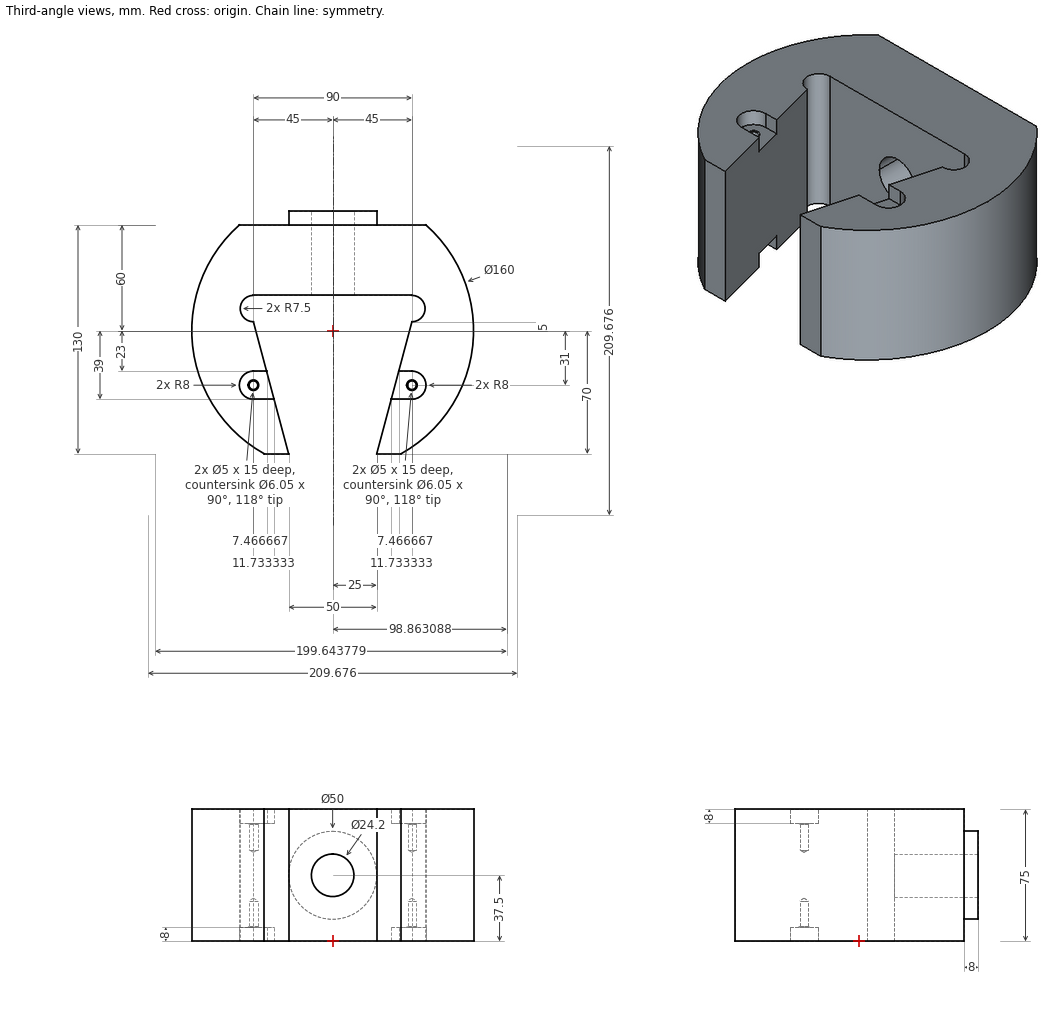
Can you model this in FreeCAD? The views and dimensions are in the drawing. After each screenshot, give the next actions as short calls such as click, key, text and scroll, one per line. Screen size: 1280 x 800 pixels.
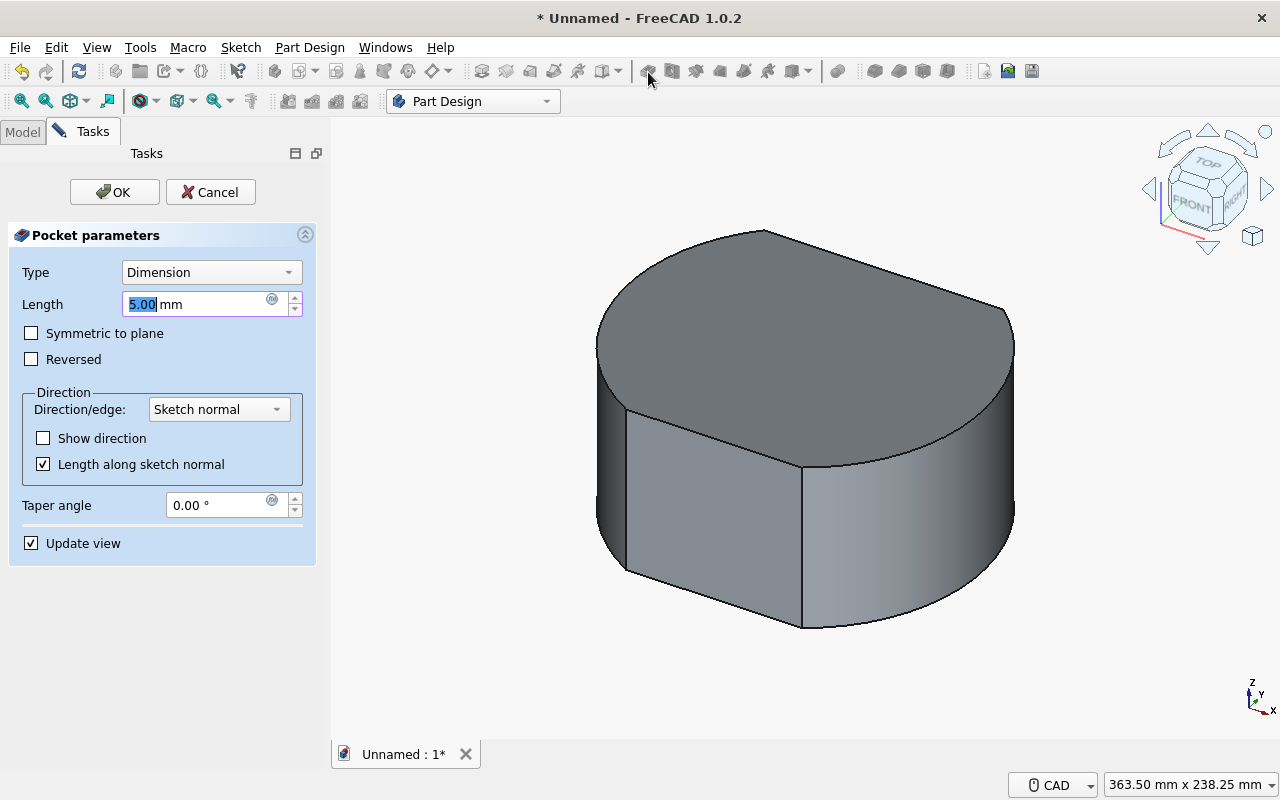
click(212, 272)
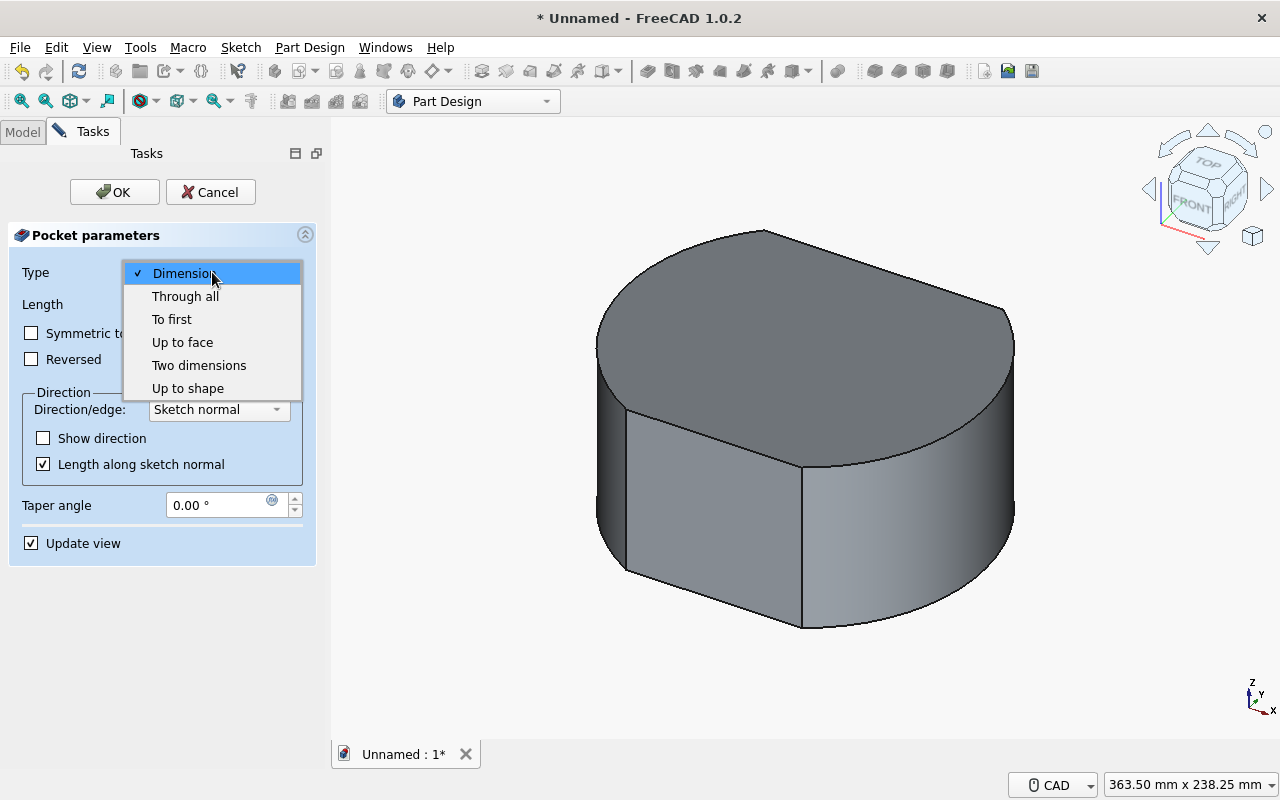
click(212, 296)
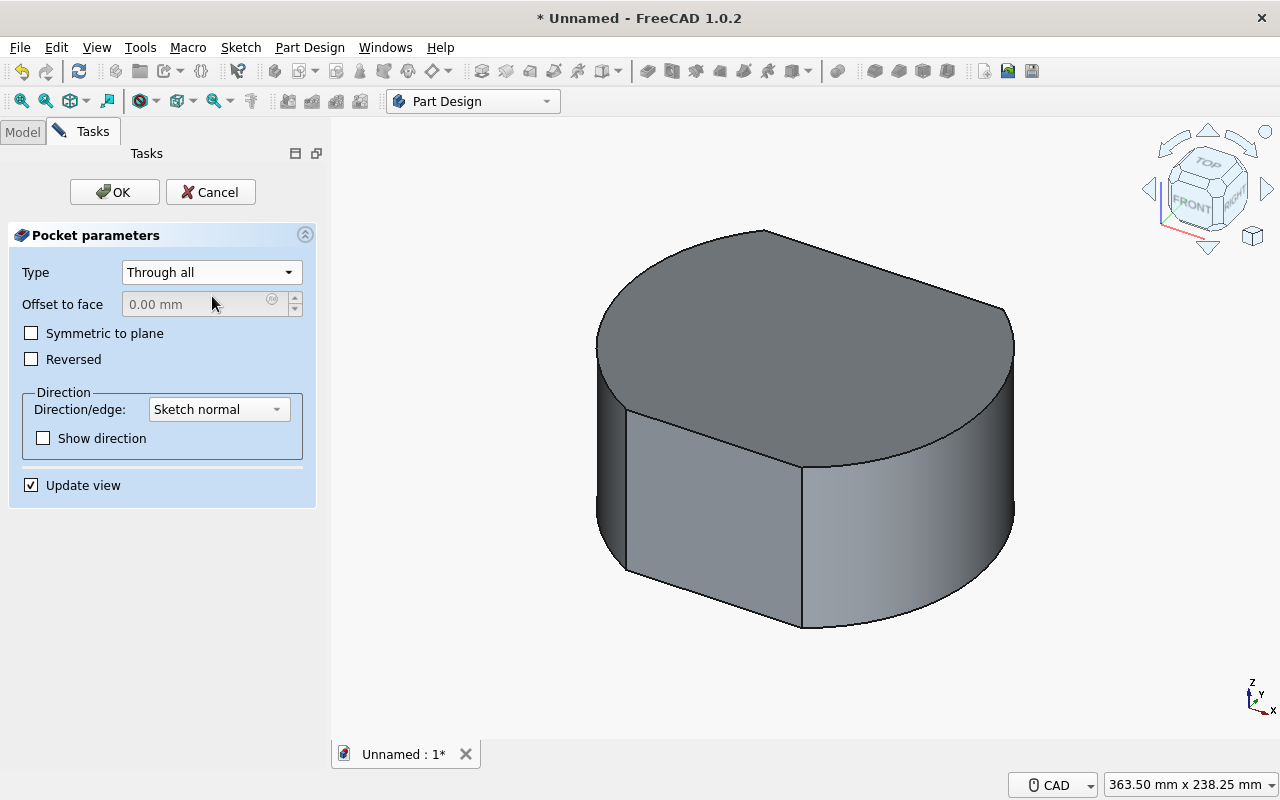
click(30, 359)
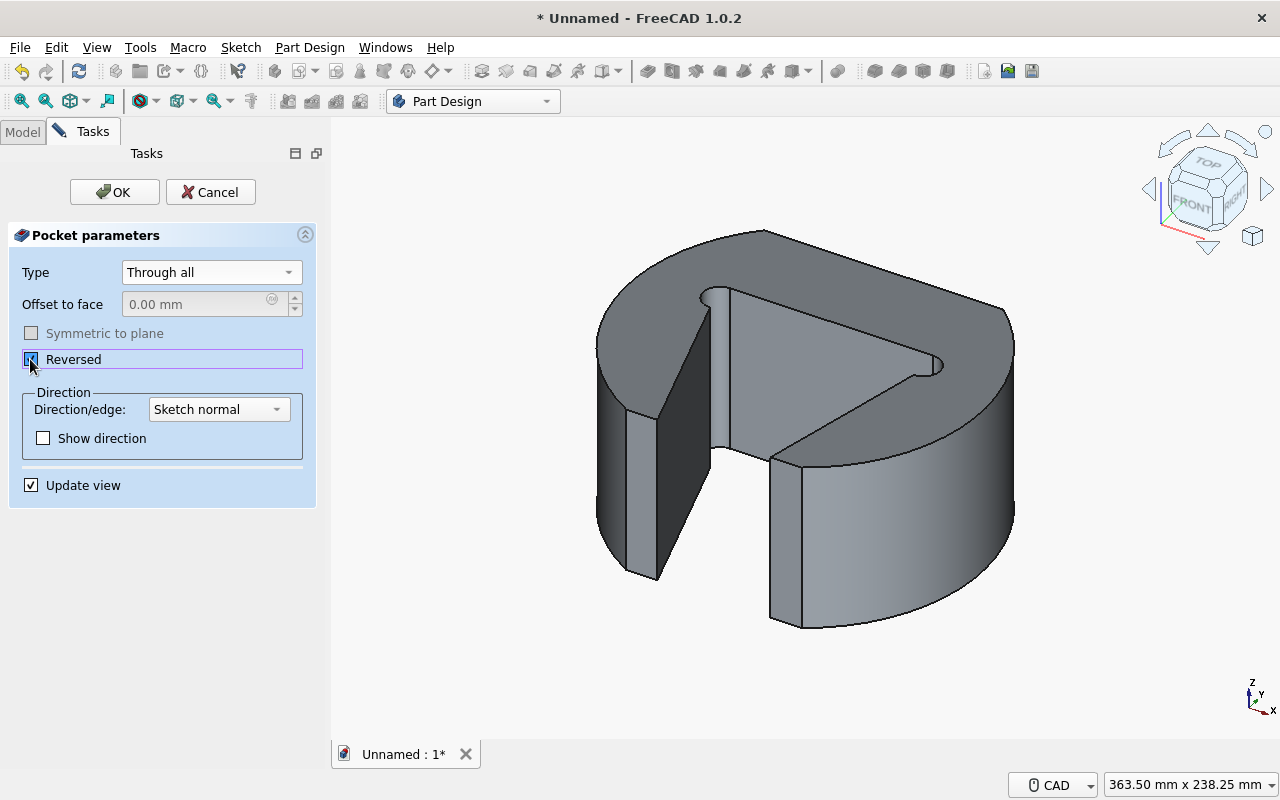
click(115, 192)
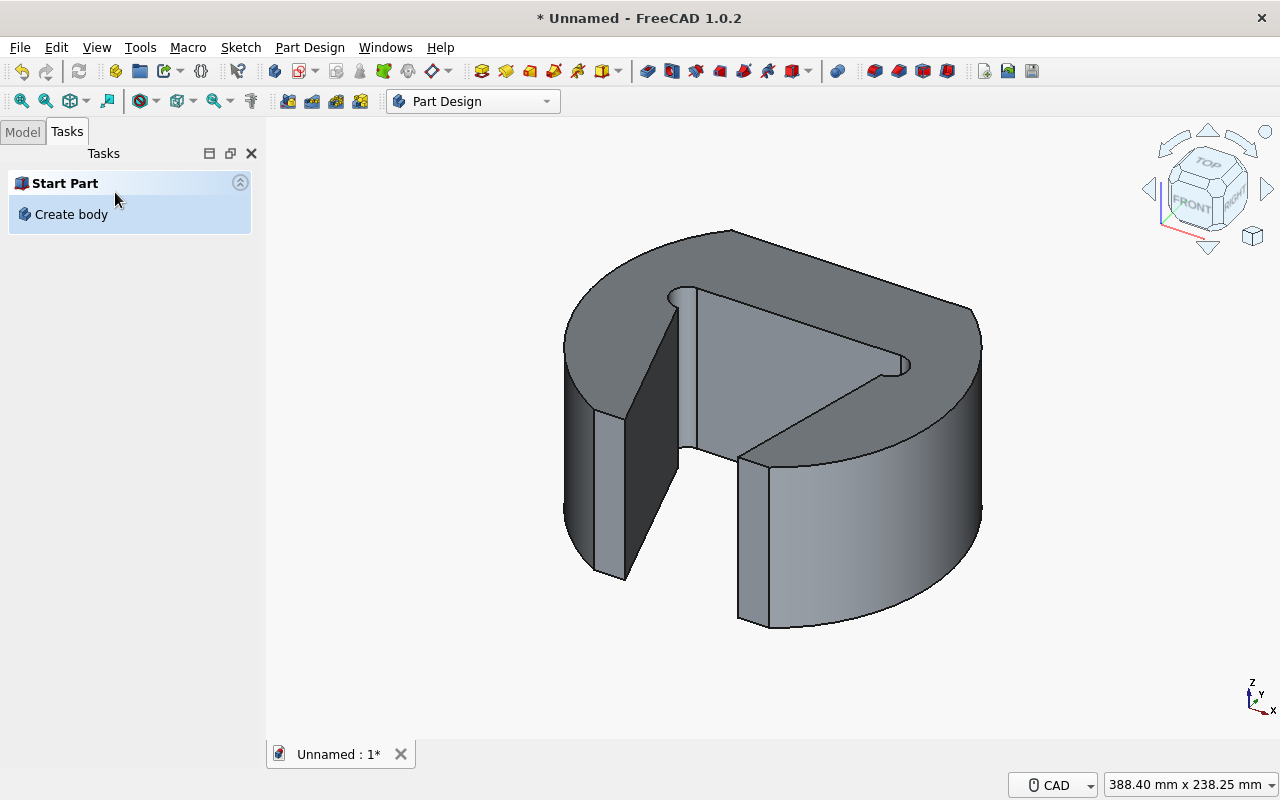
key(5)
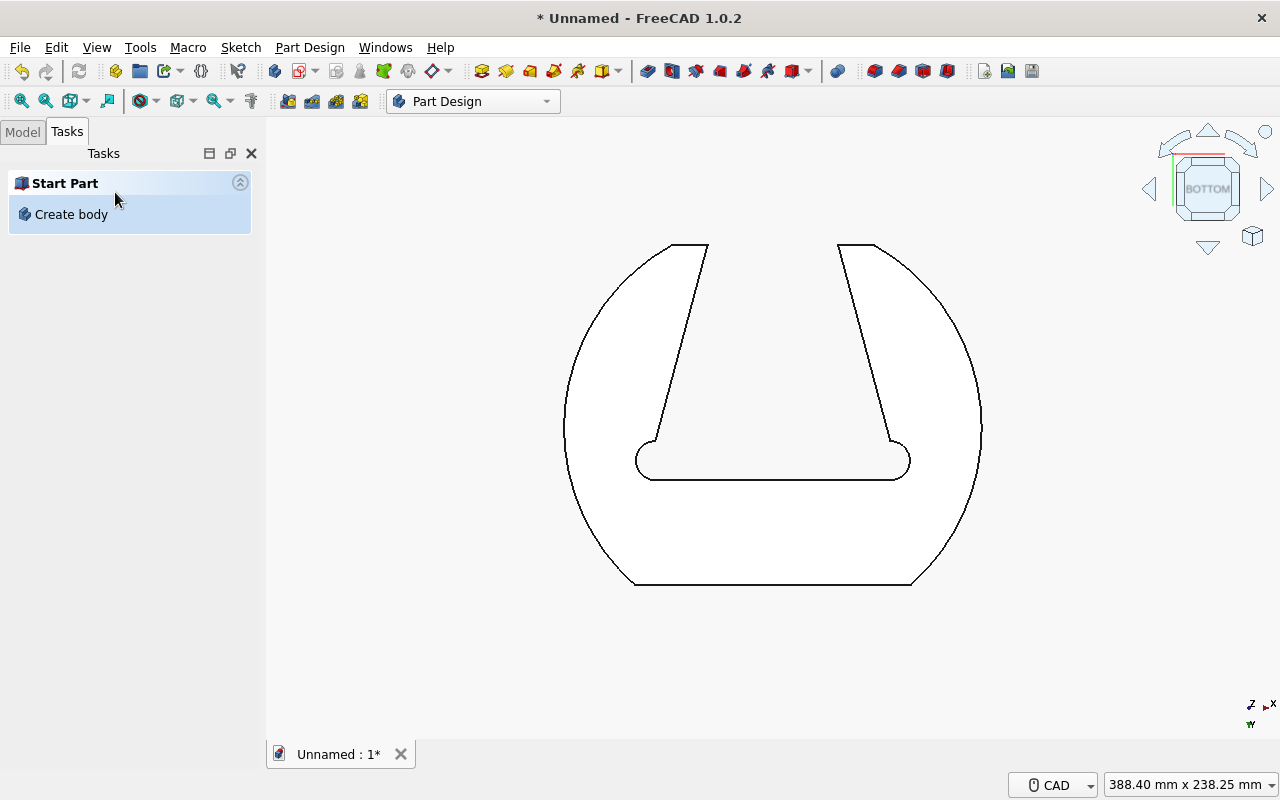
click(653, 317)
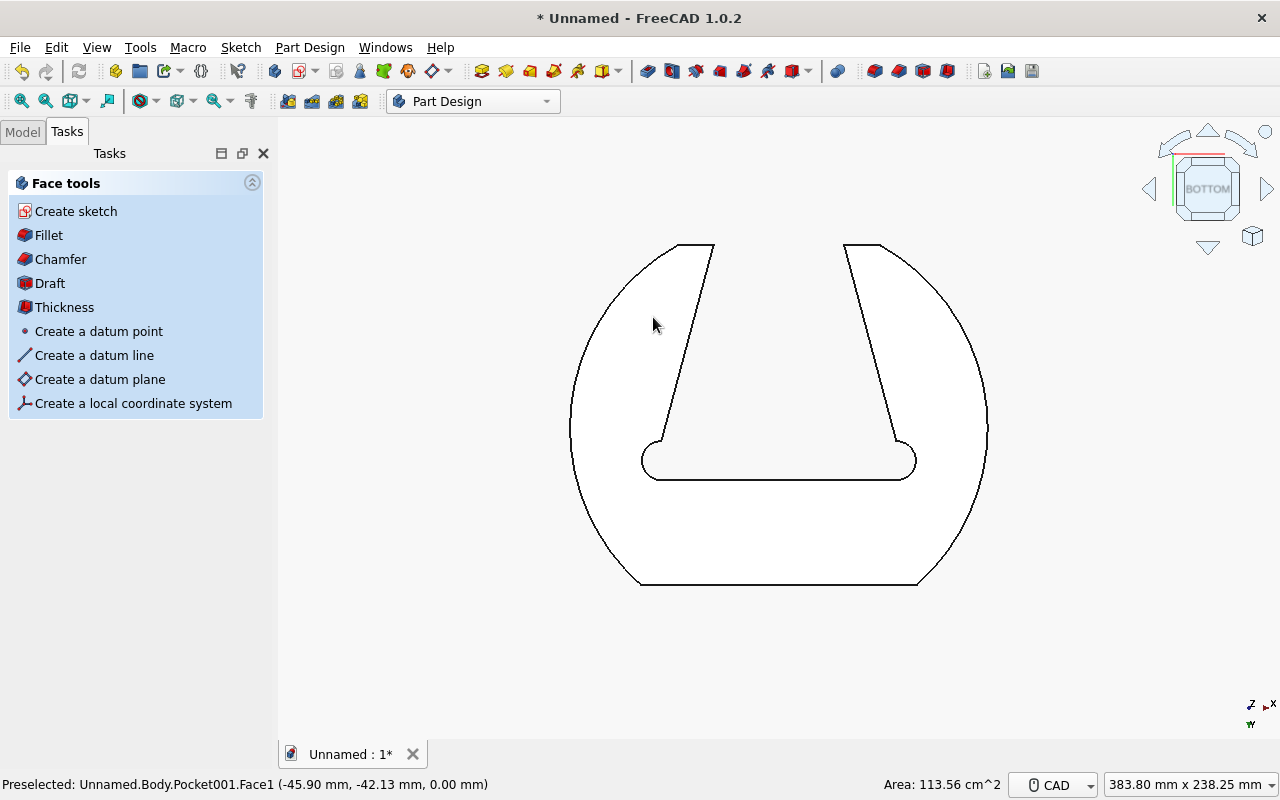
click(300, 72)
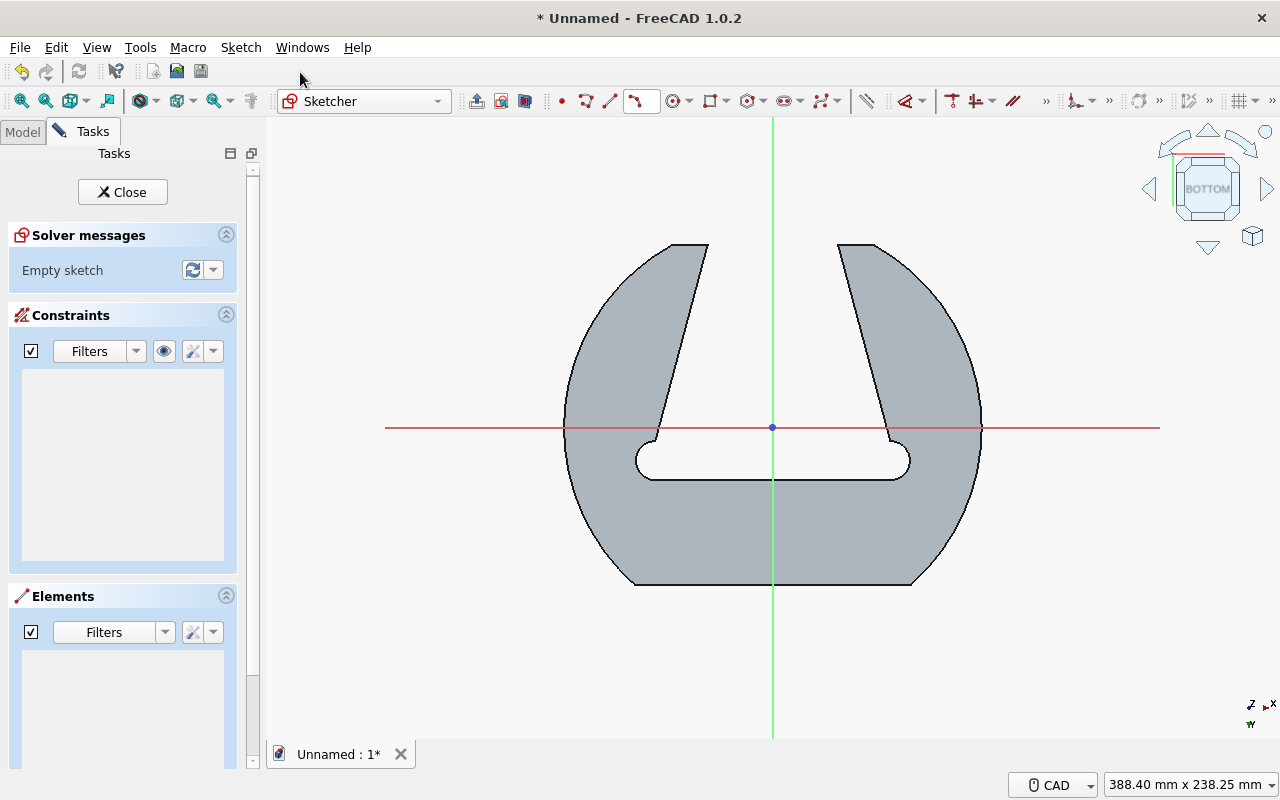
scroll(829, 336, up, 4)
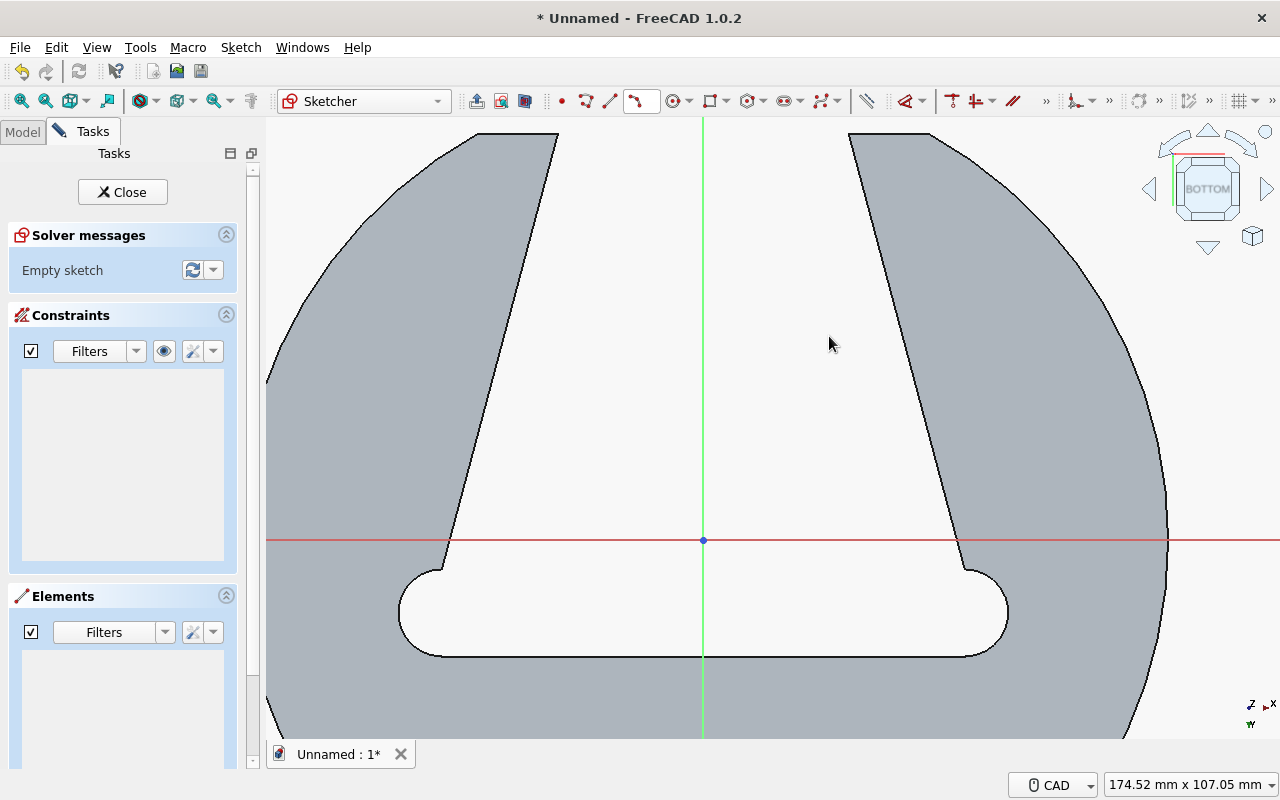
key(g)
key(s)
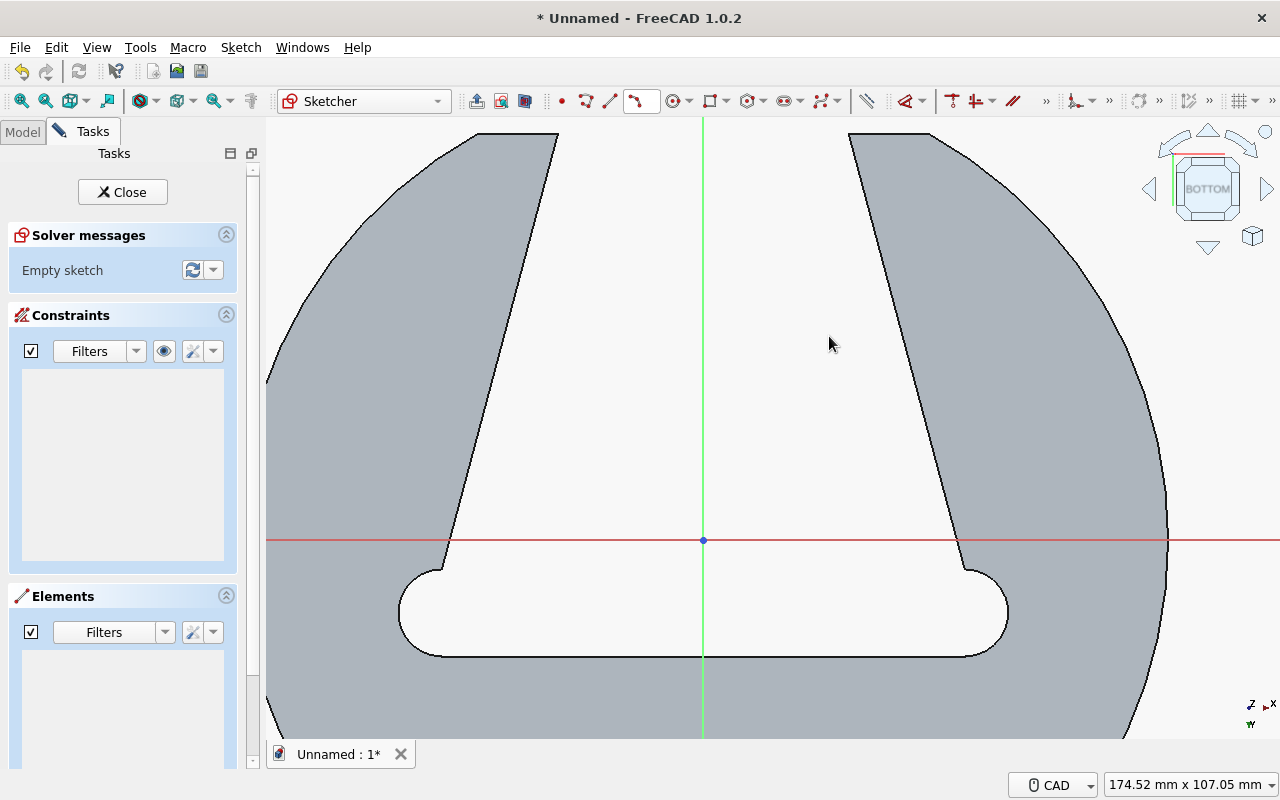
click(442, 360)